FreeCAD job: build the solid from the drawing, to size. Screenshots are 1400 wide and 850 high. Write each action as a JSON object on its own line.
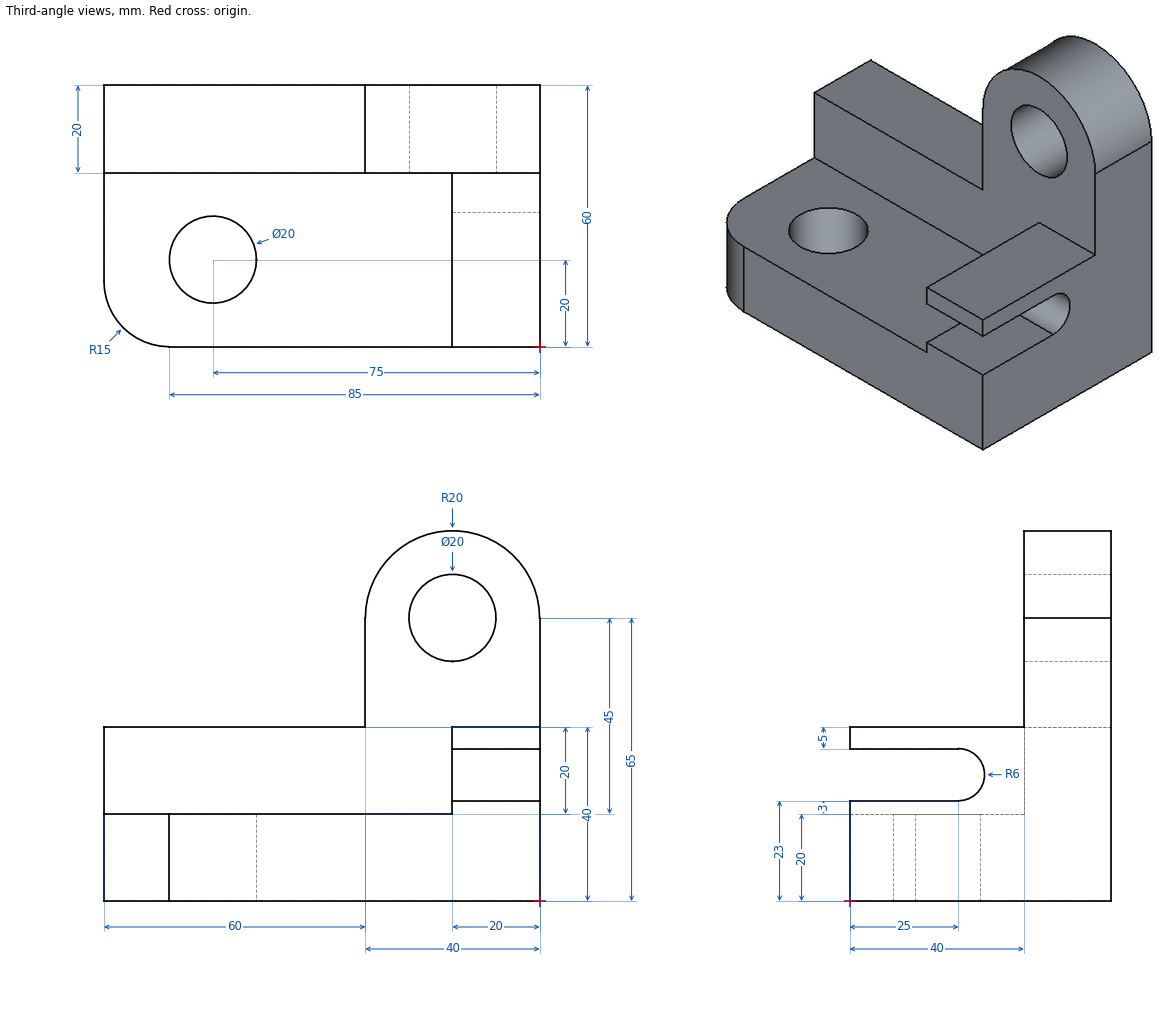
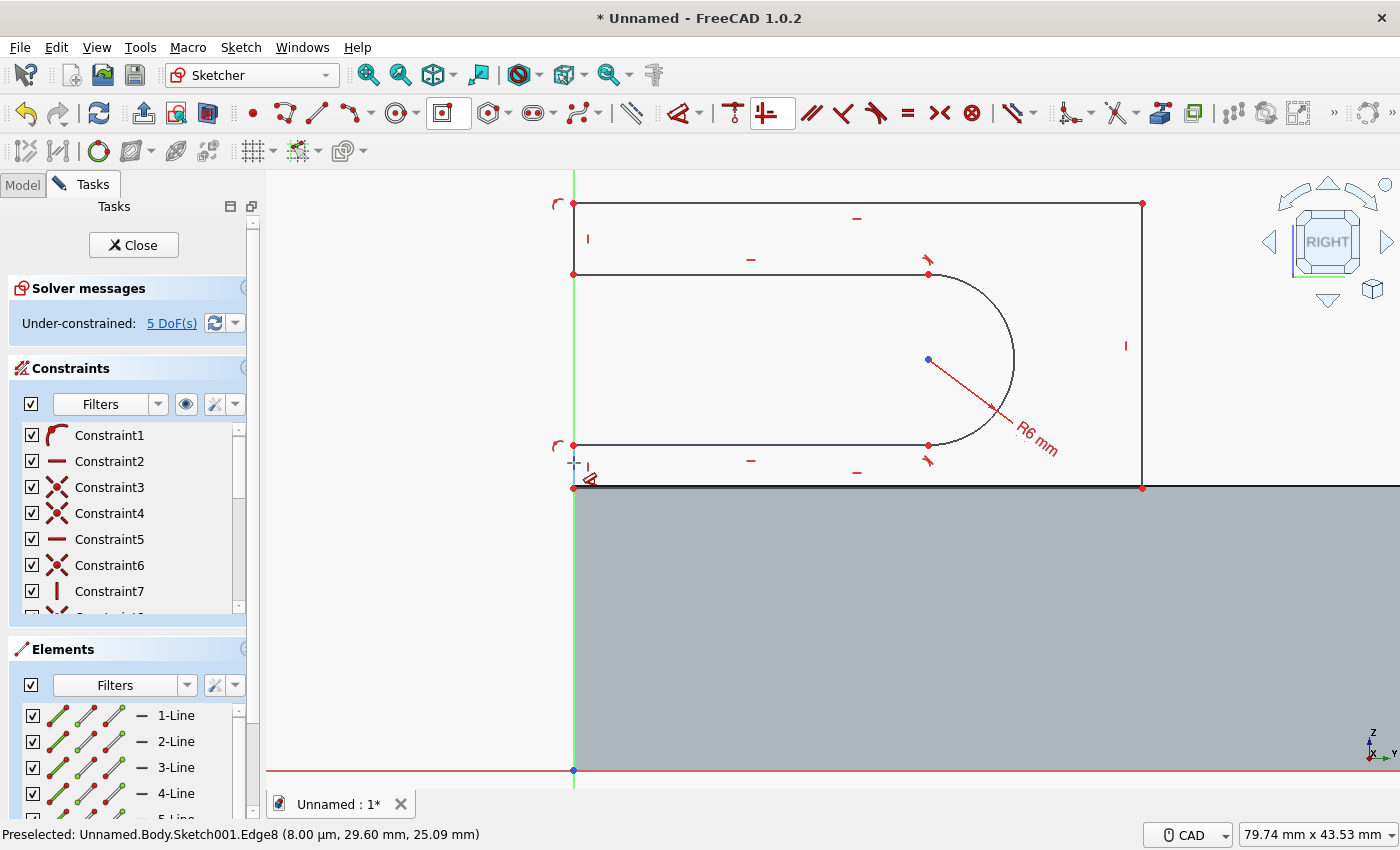
{"action": "left_click", "coordinate": [574, 462]}
{"action": "left_click", "coordinate": [540, 467]}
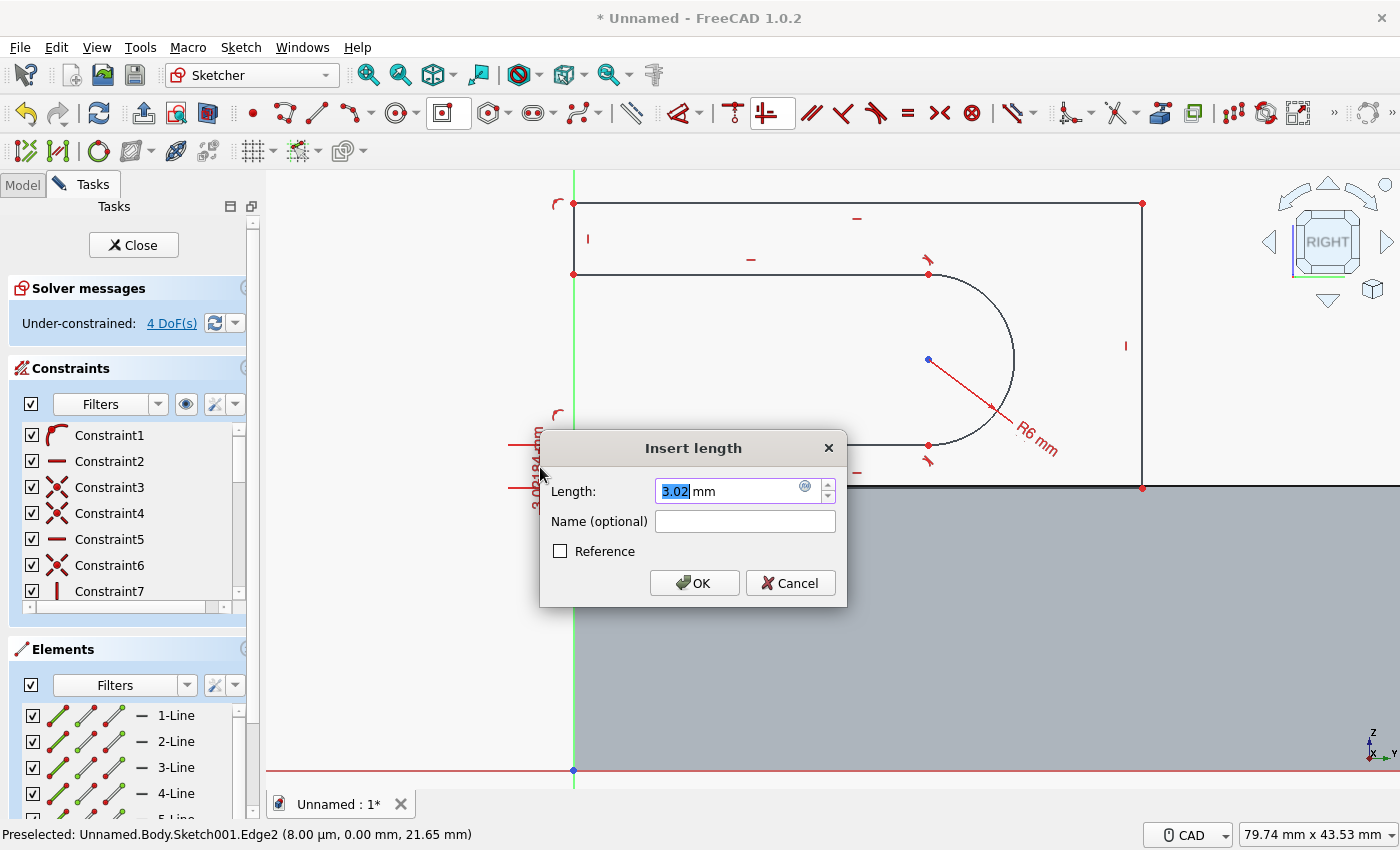
{"action": "type", "text": "3"}
{"action": "key", "text": "Return"}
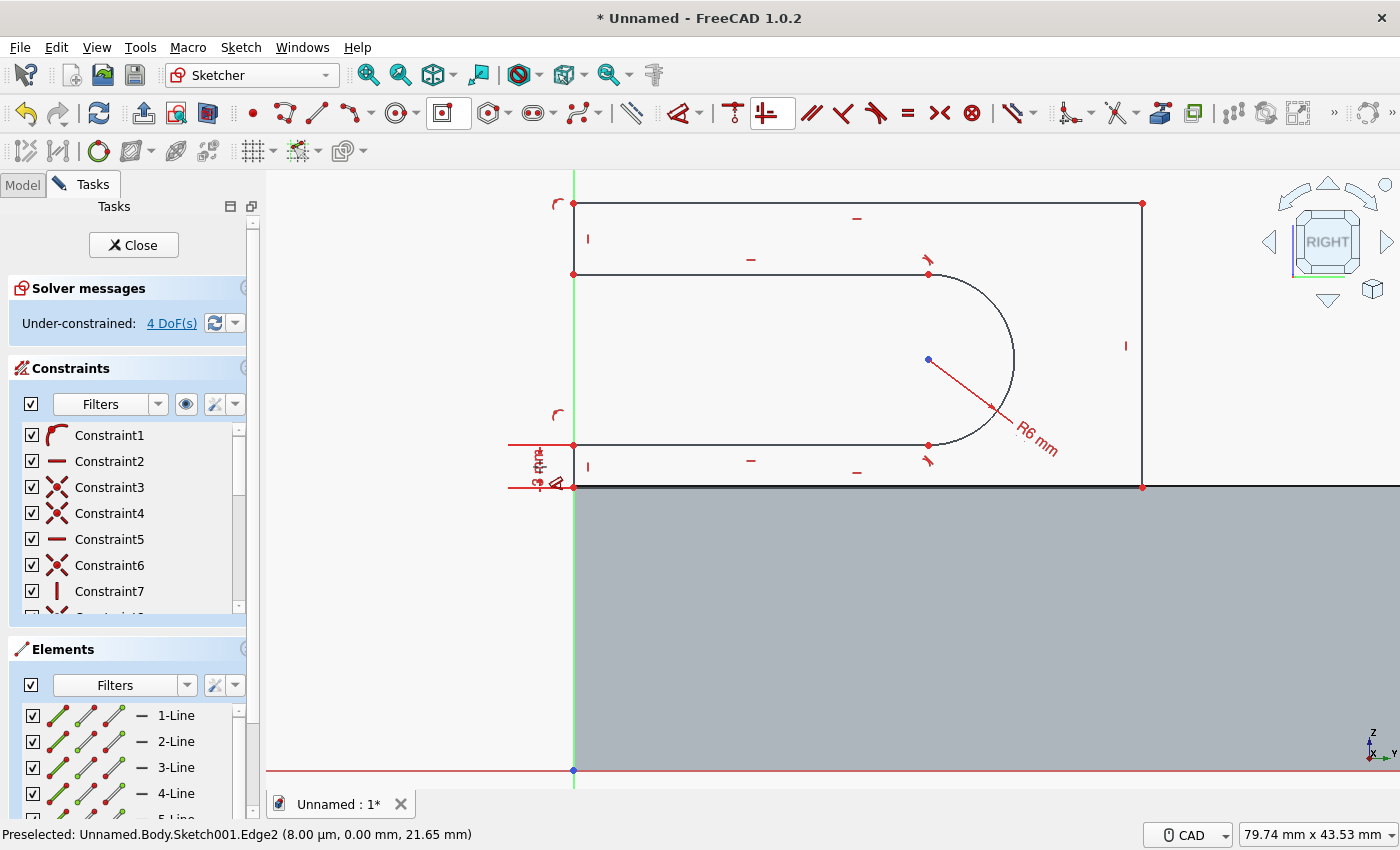
{"action": "left_click", "coordinate": [574, 225]}
{"action": "left_click", "coordinate": [540, 239]}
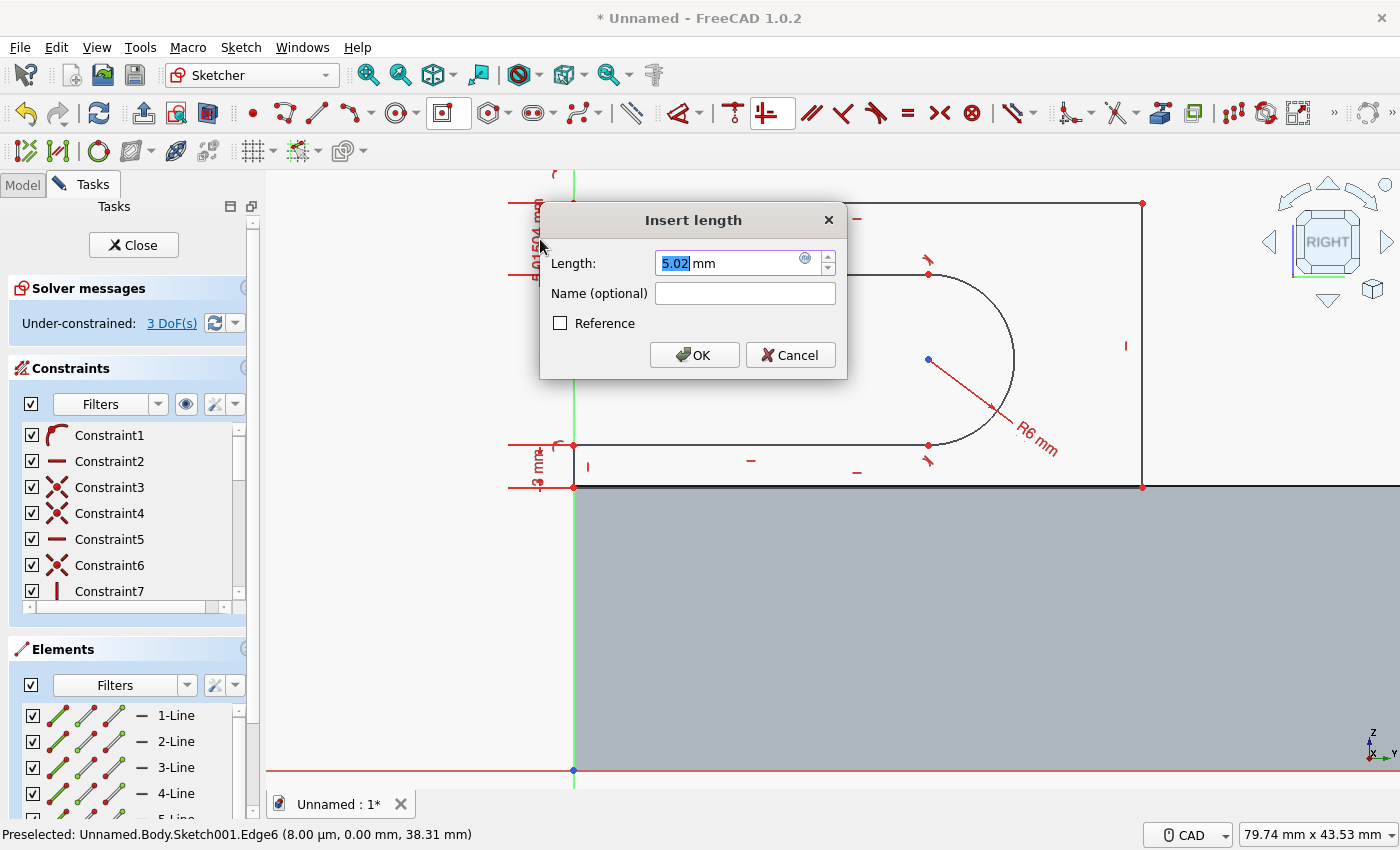
{"action": "type", "text": "5"}
{"action": "key", "text": "Return"}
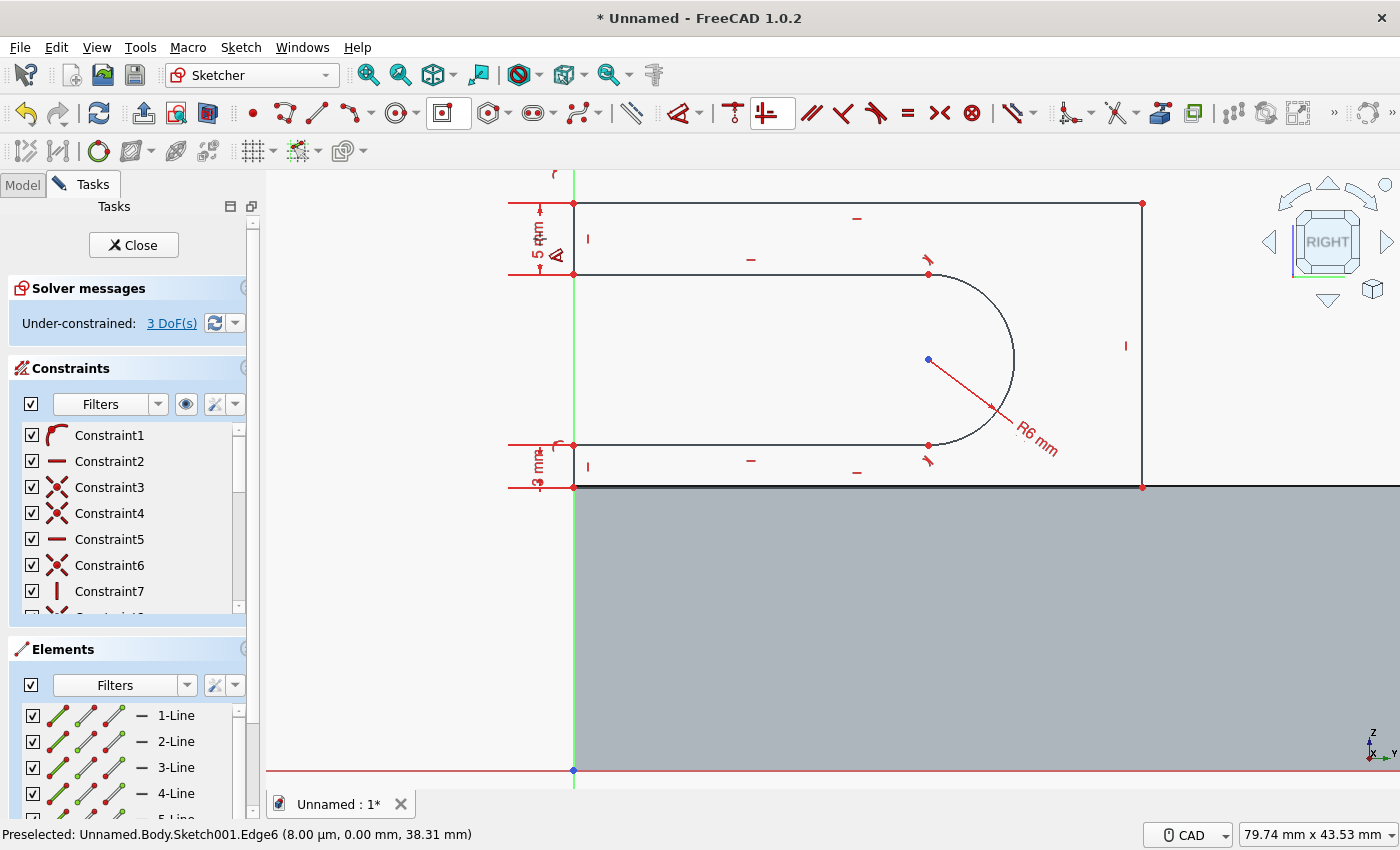
{"action": "left_click", "coordinate": [822, 445]}
{"action": "left_click", "coordinate": [751, 411]}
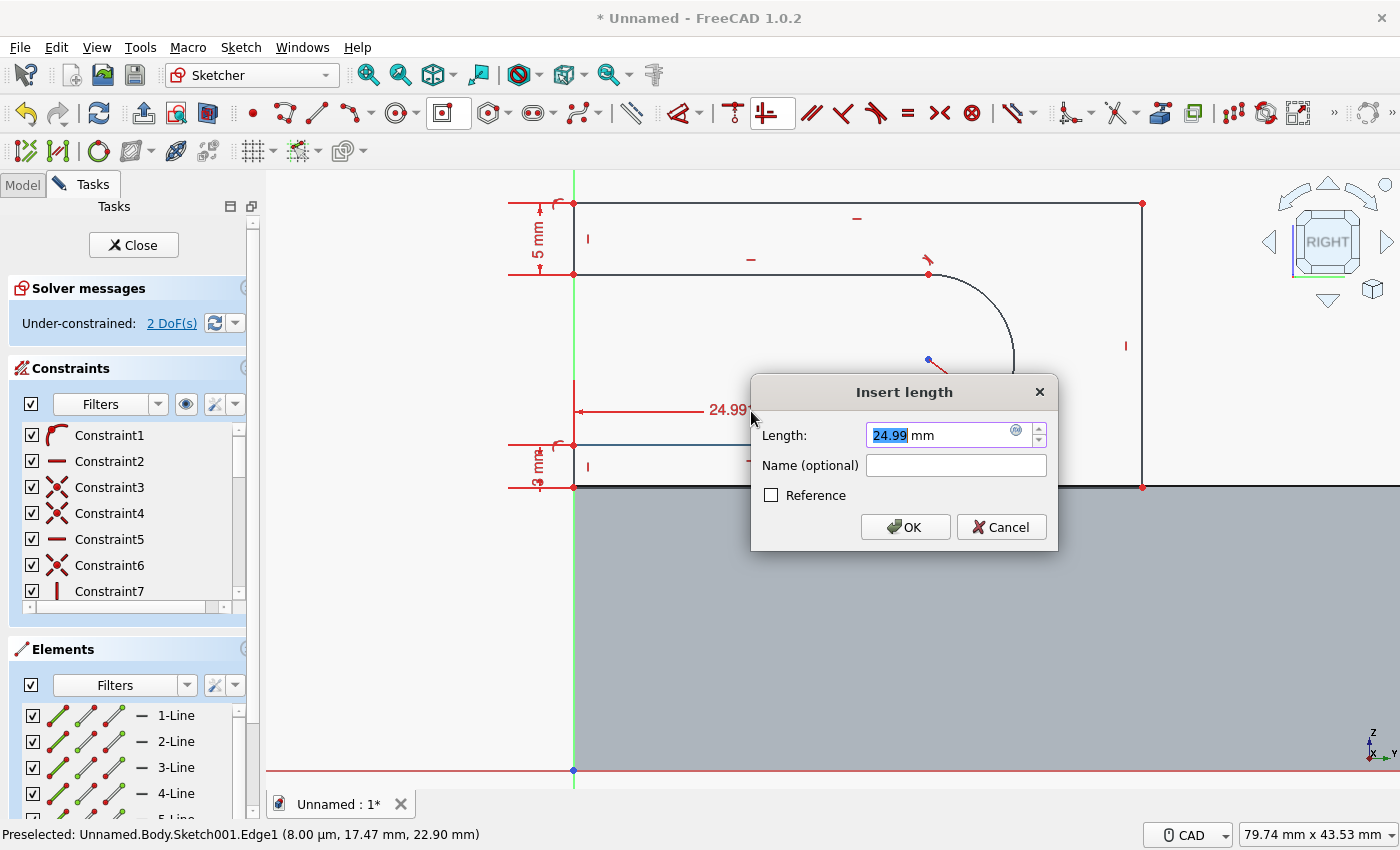
{"action": "type", "text": "25"}
{"action": "key", "text": "Return"}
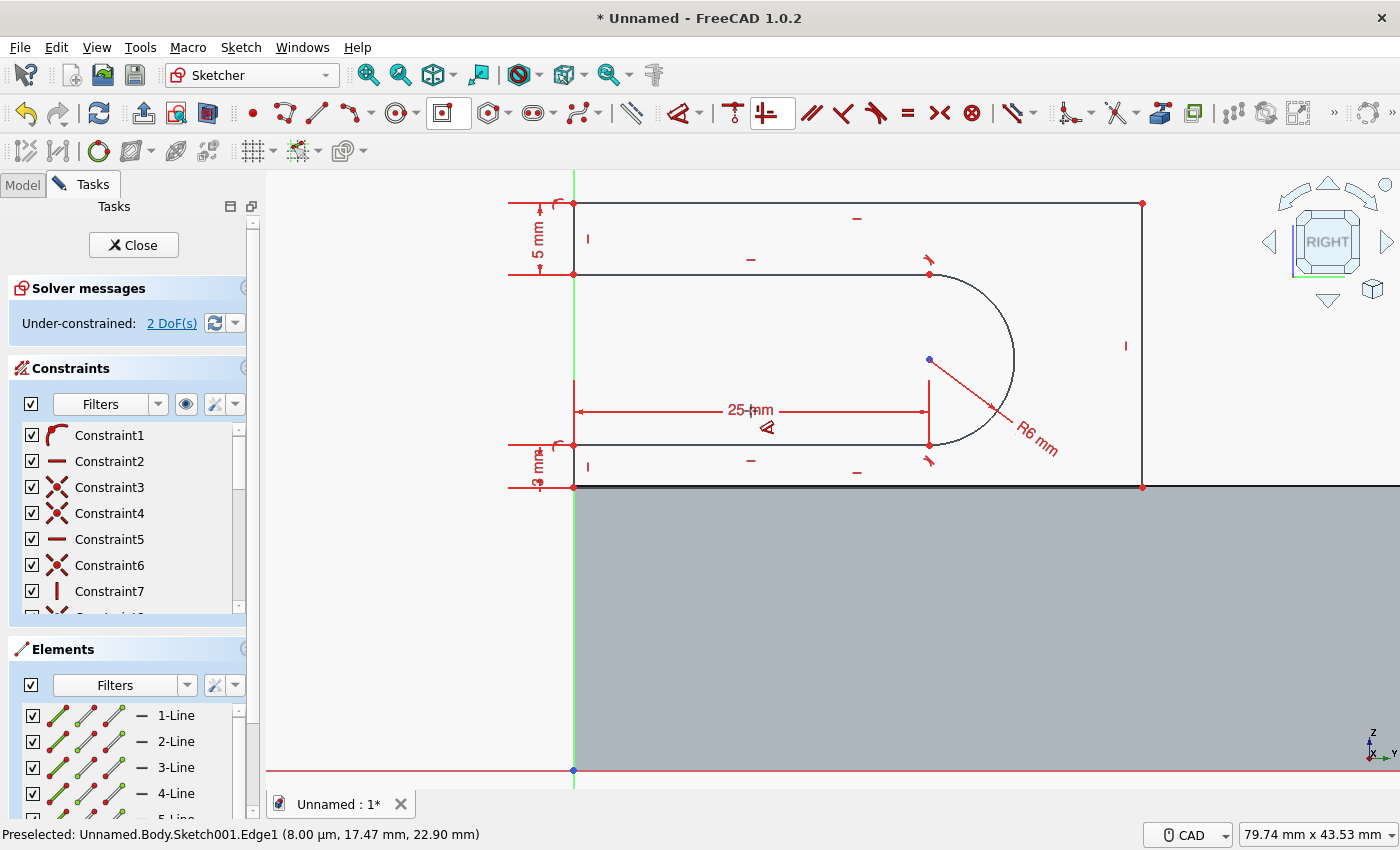
{"action": "left_click", "coordinate": [744, 488]}
{"action": "left_click", "coordinate": [858, 522]}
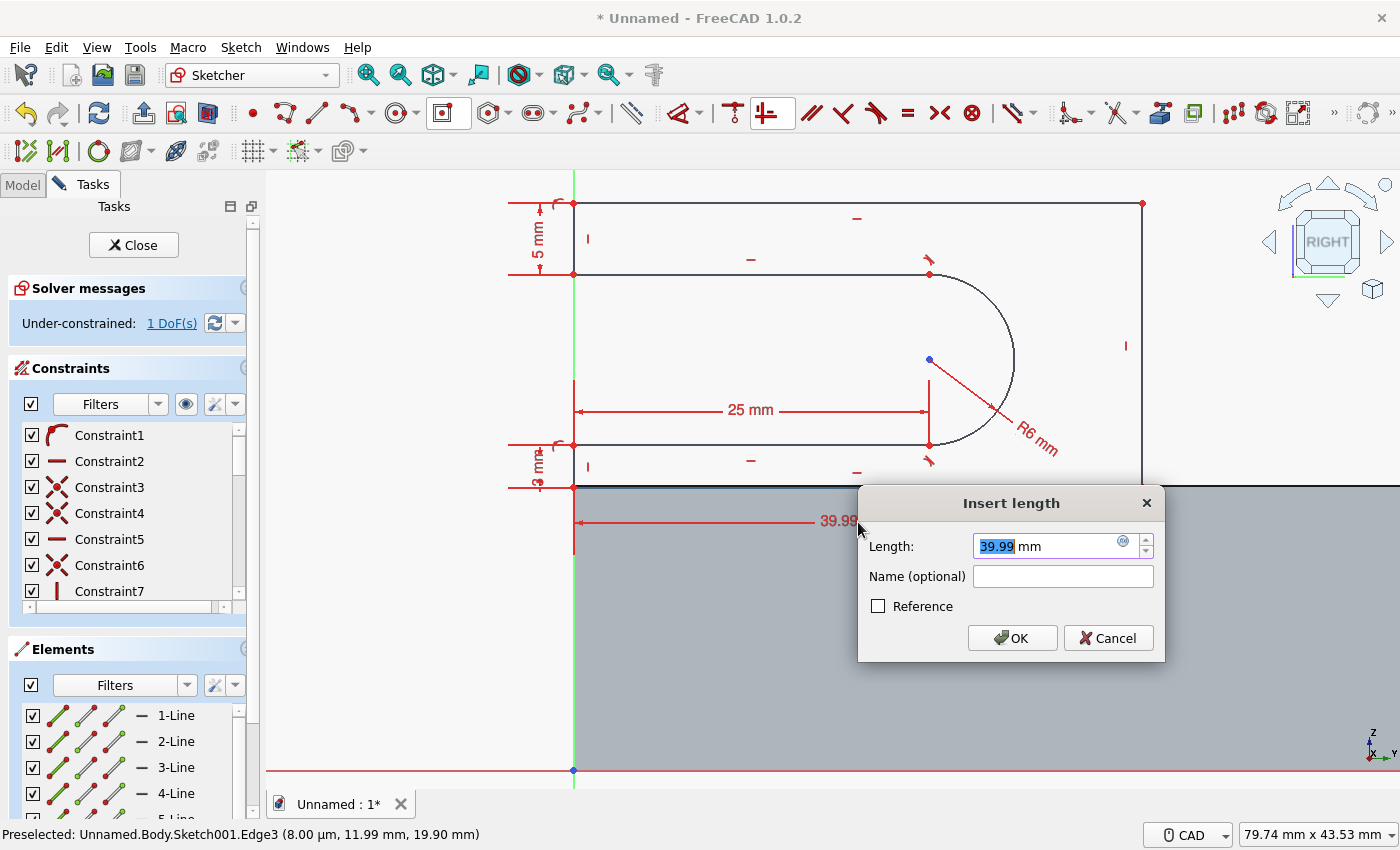
{"action": "type", "text": "40"}
{"action": "key", "text": "Return"}